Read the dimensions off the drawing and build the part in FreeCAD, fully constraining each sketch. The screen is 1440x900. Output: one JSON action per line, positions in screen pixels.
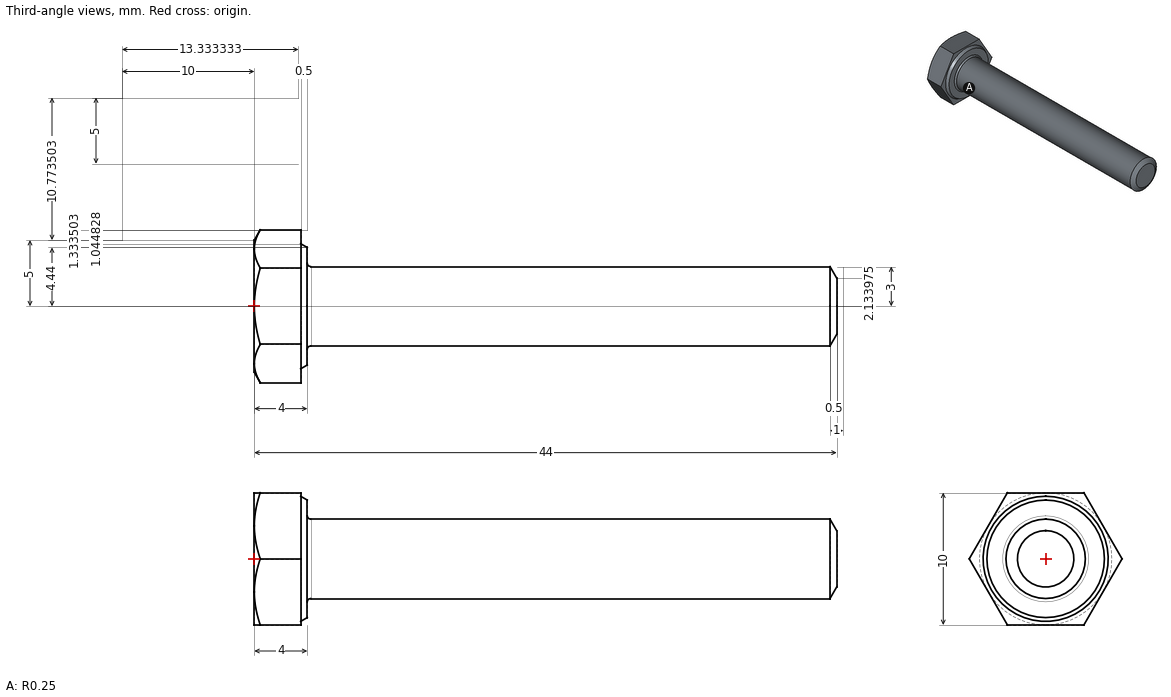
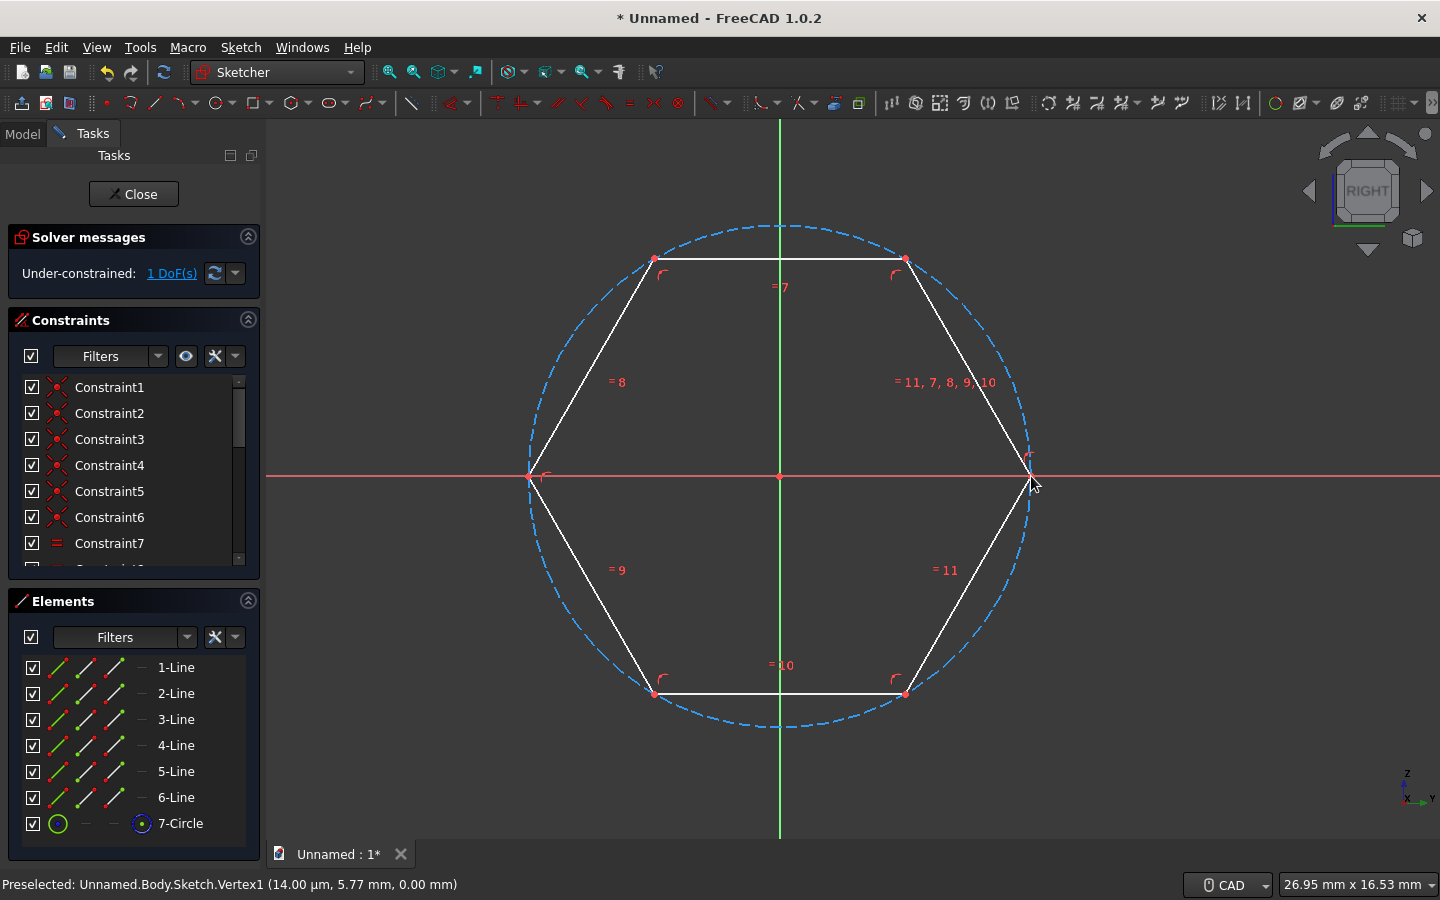
{"action": "left_click", "coordinate": [654, 694]}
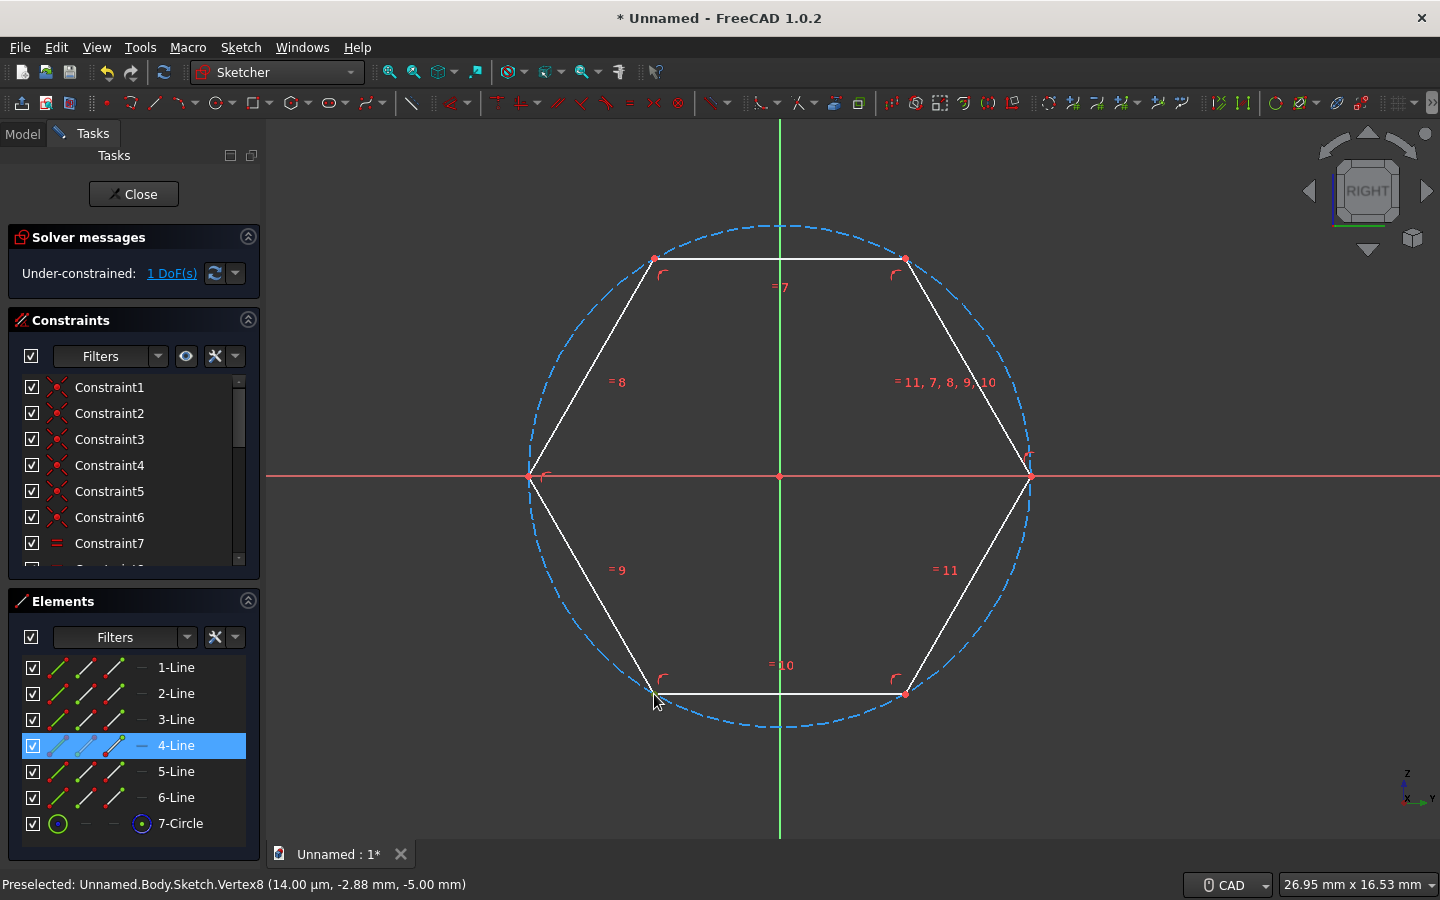
{"action": "left_click", "coordinate": [905, 259]}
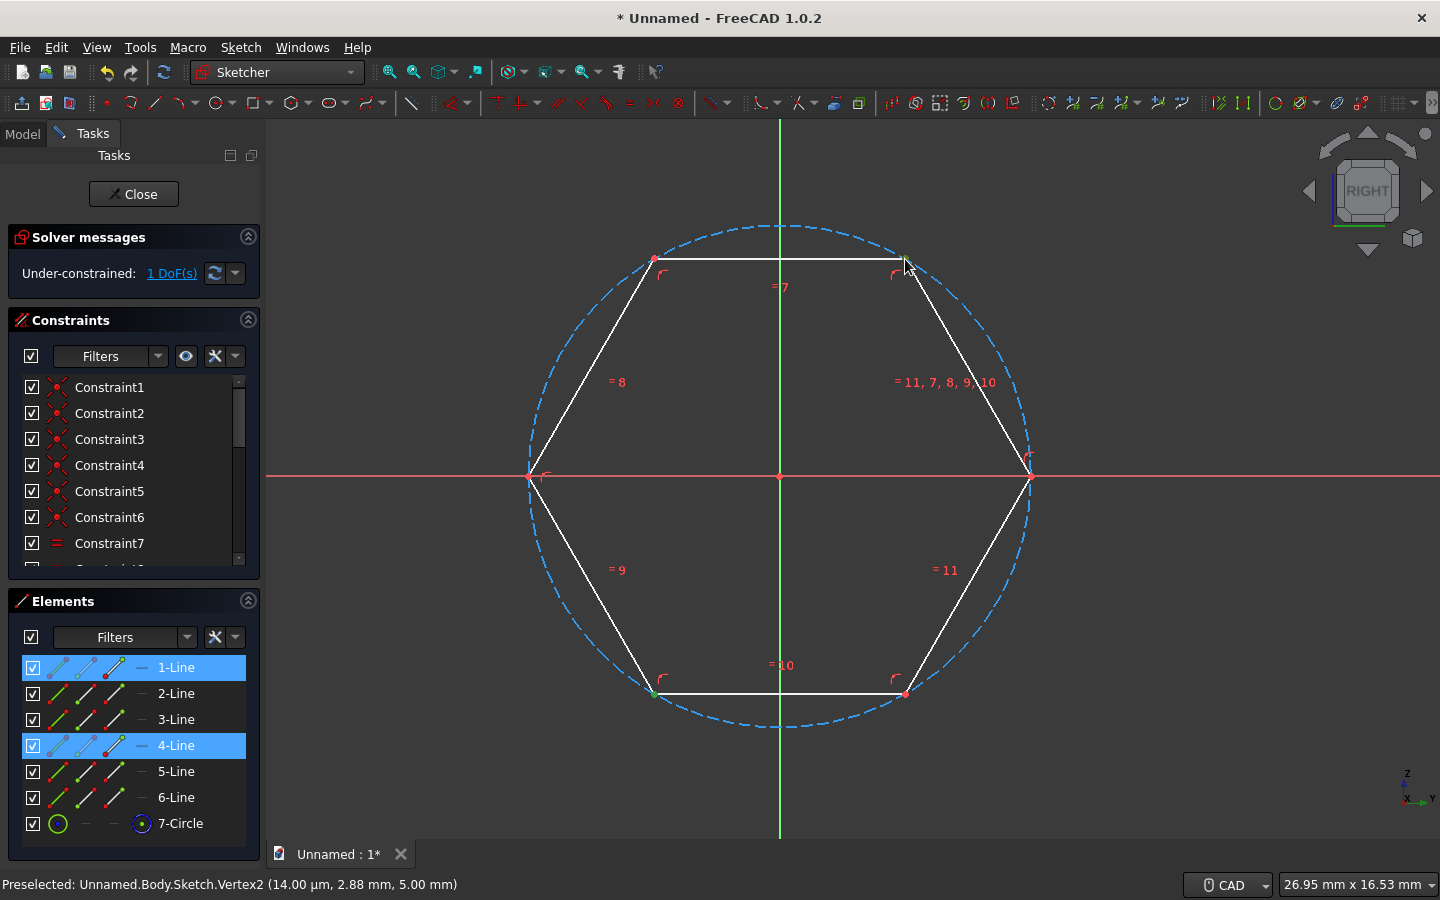
{"action": "left_click", "coordinate": [470, 104]}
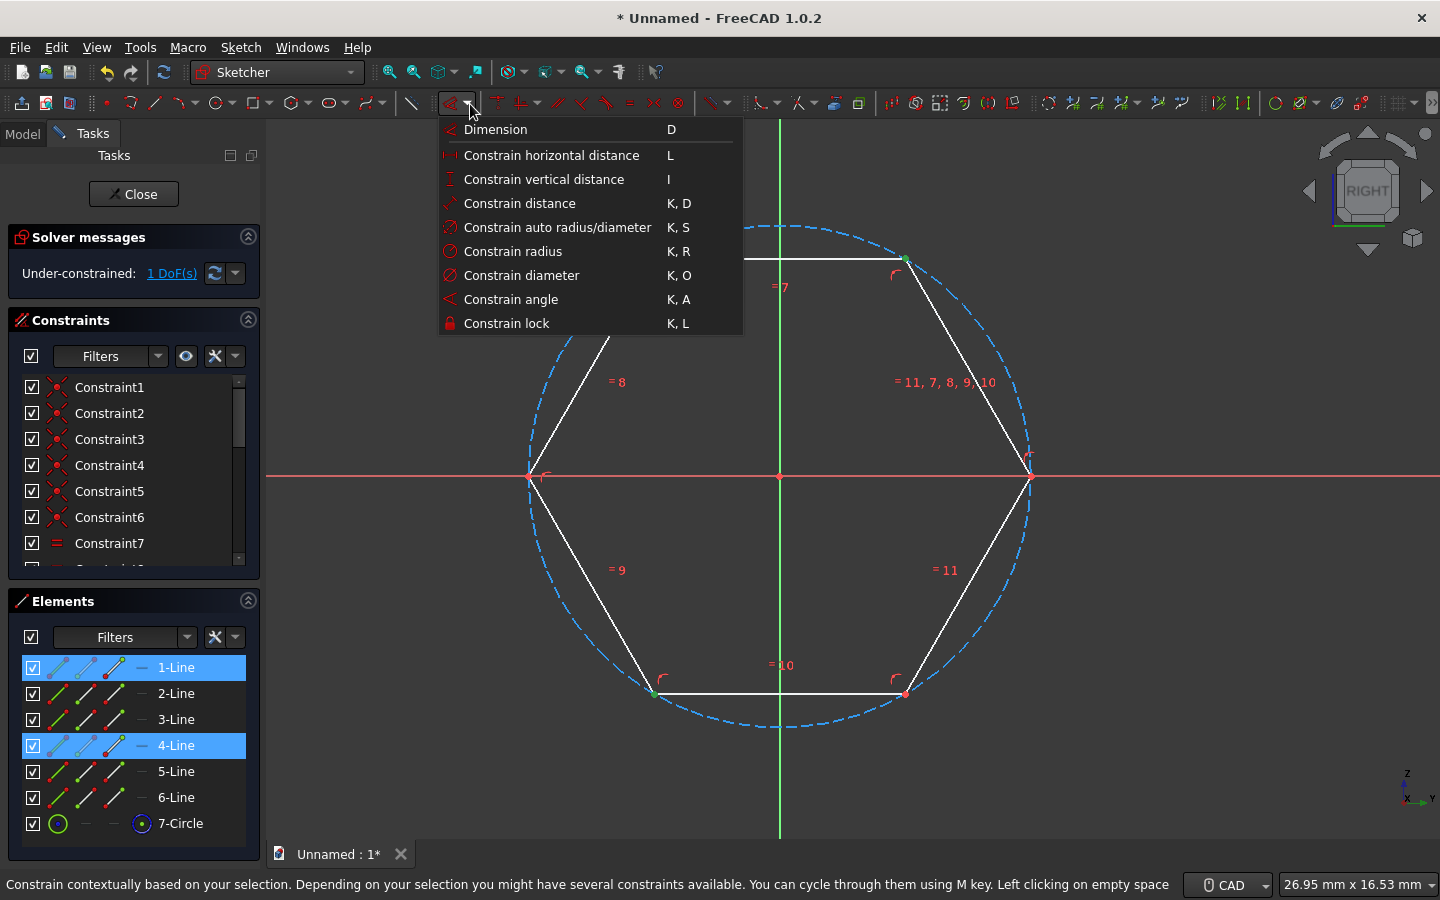
{"action": "left_click", "coordinate": [591, 179]}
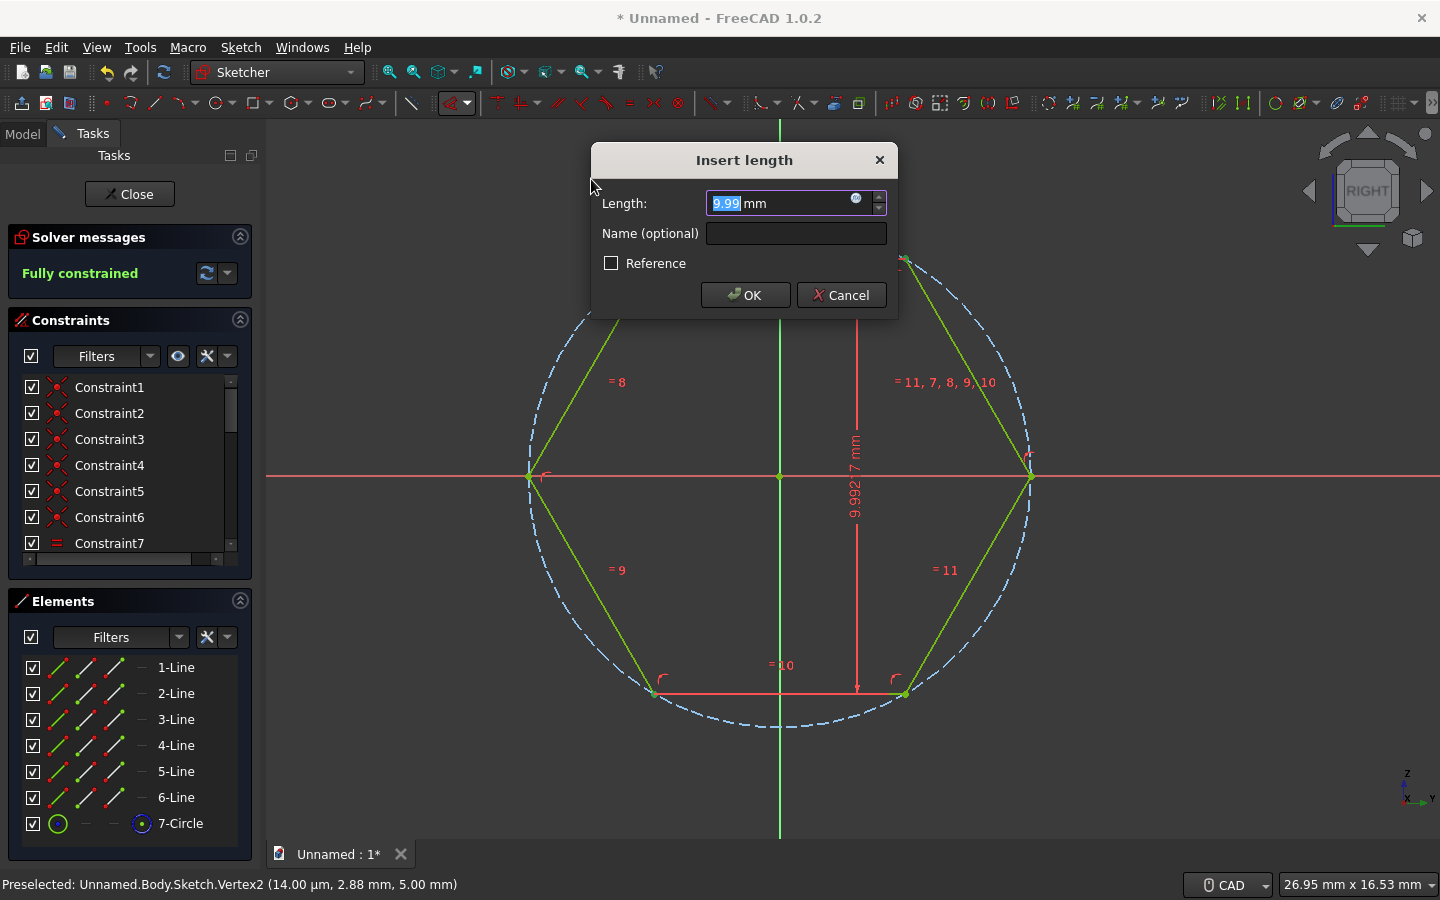
{"action": "type", "text": "10"}
{"action": "key", "text": "Return"}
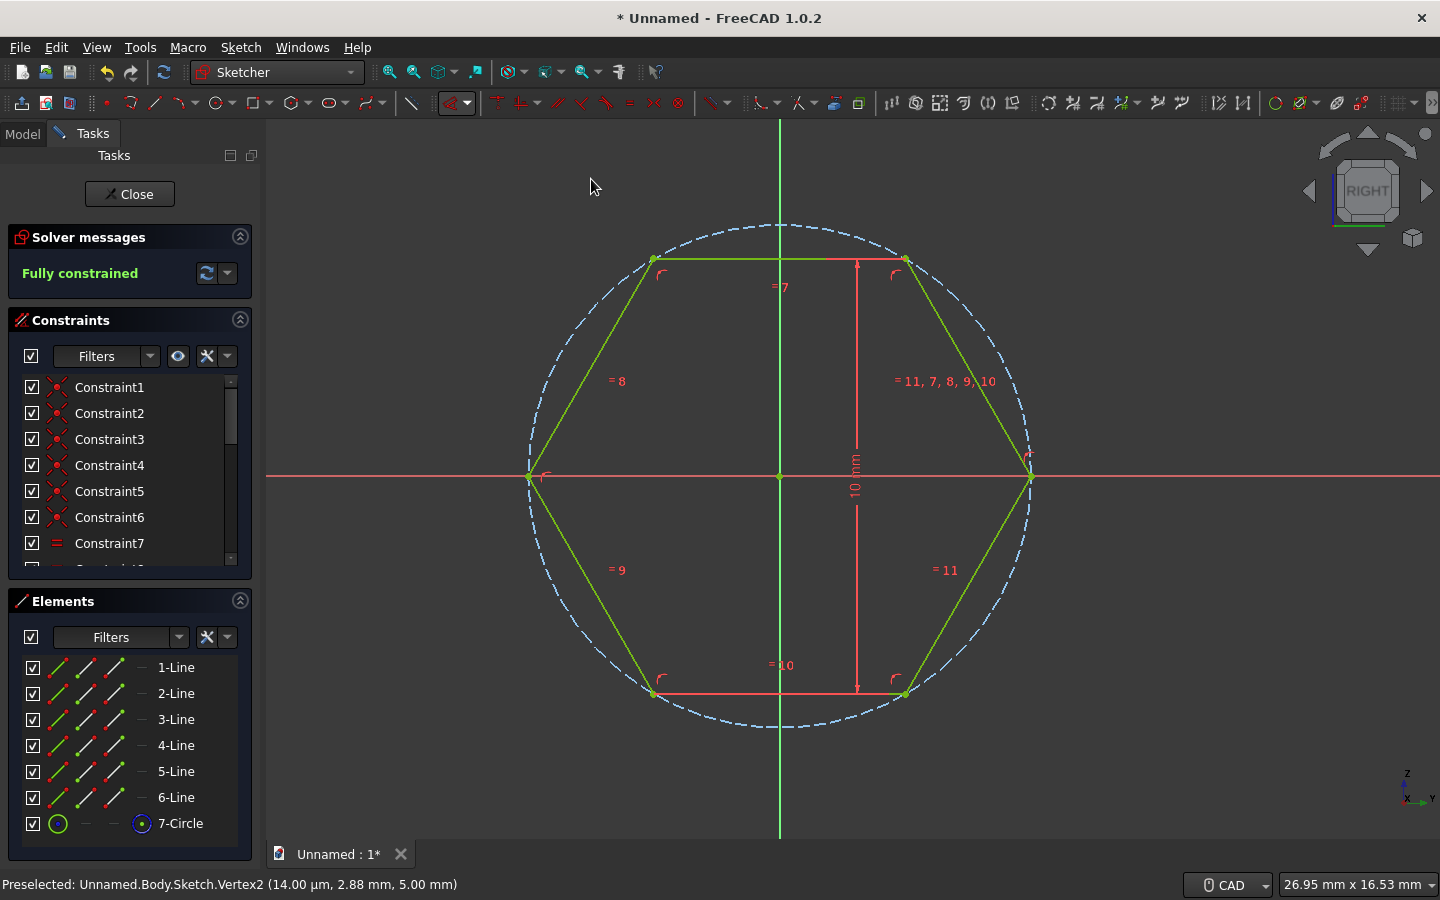
{"action": "left_click", "coordinate": [130, 194]}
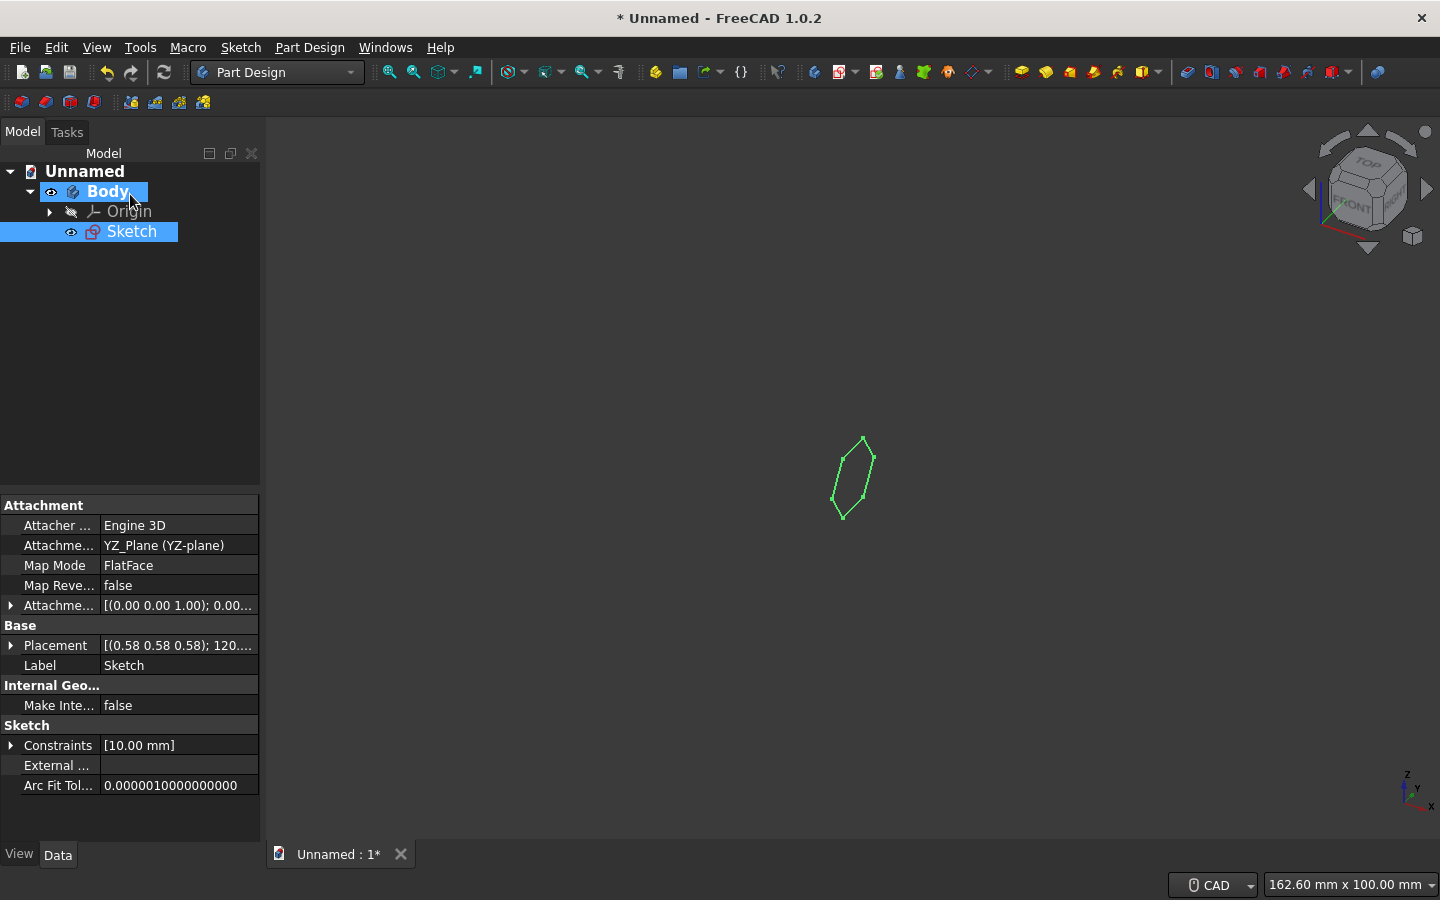
{"action": "left_click", "coordinate": [1022, 72]}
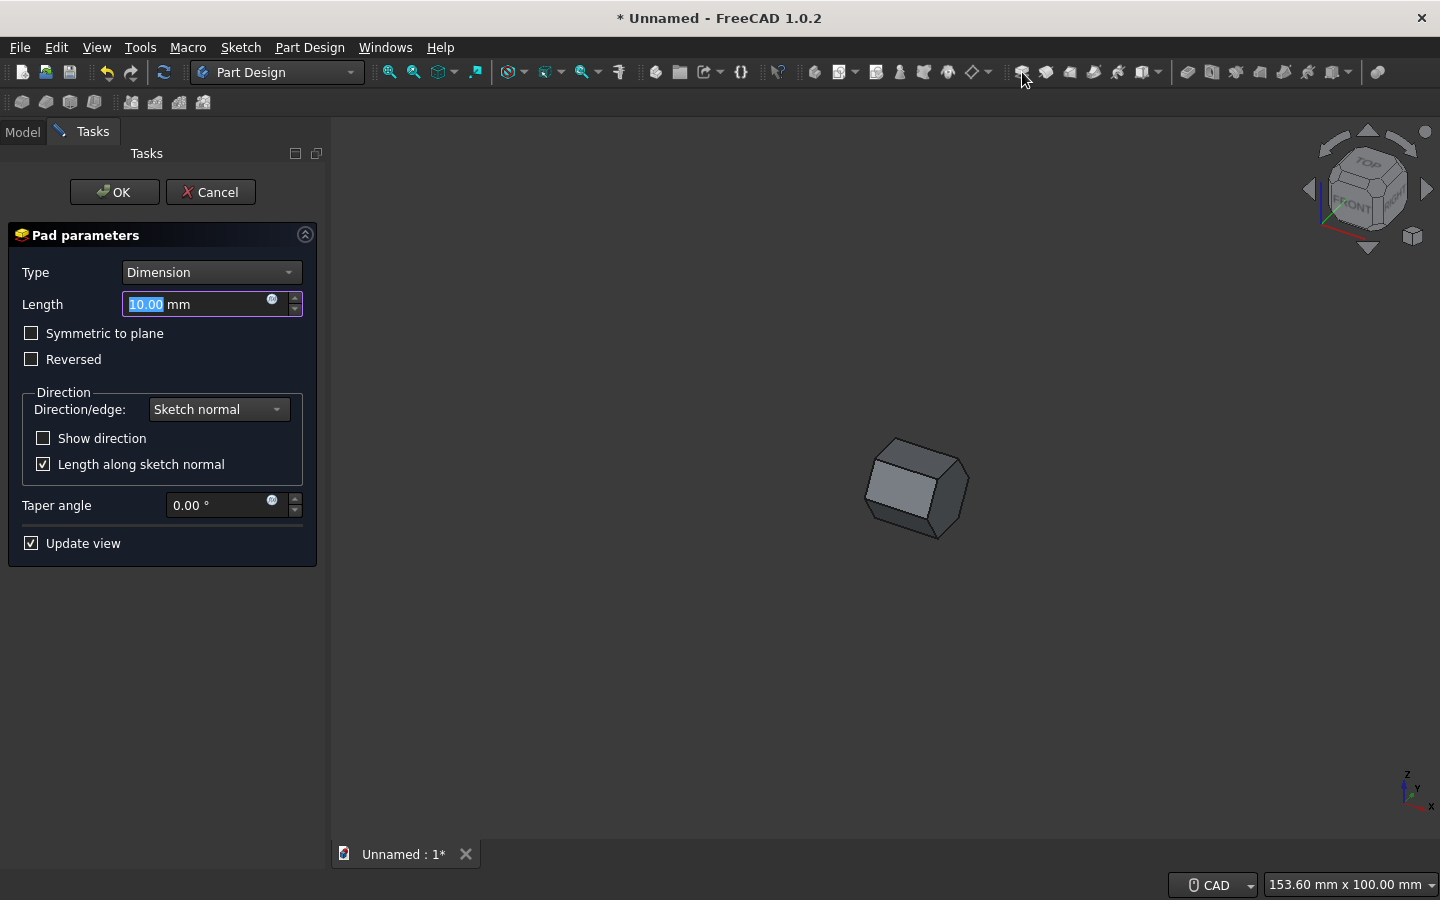
{"action": "type", "text": "4"}
{"action": "key", "text": "Tab"}